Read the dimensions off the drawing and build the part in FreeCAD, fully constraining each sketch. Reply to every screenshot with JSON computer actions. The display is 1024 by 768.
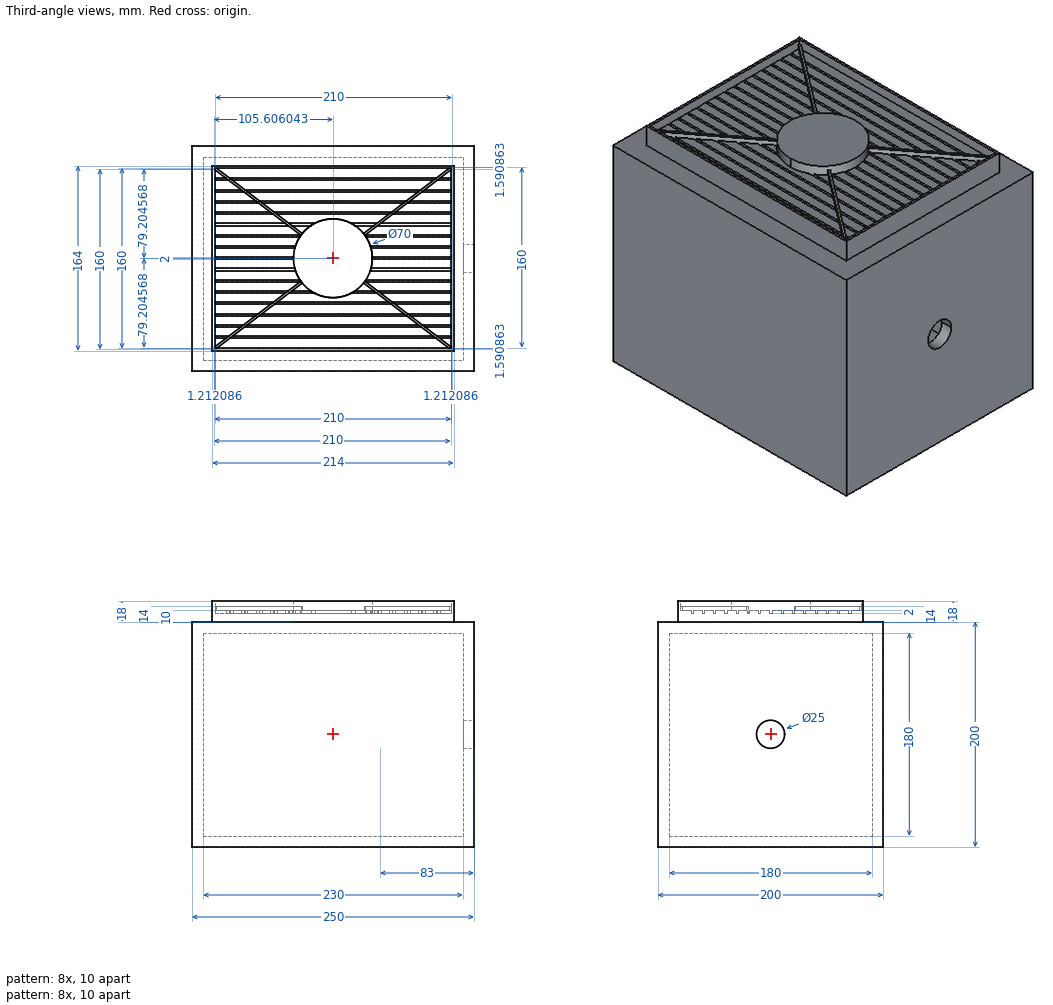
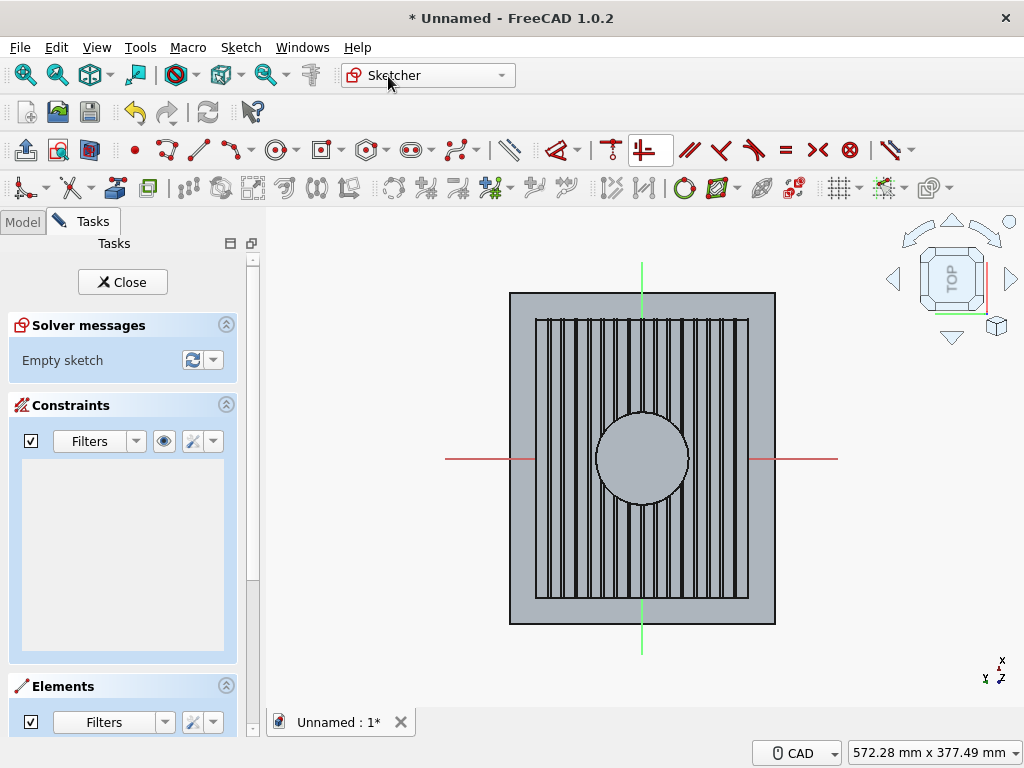
{"action": "left_click", "coordinate": [90, 150]}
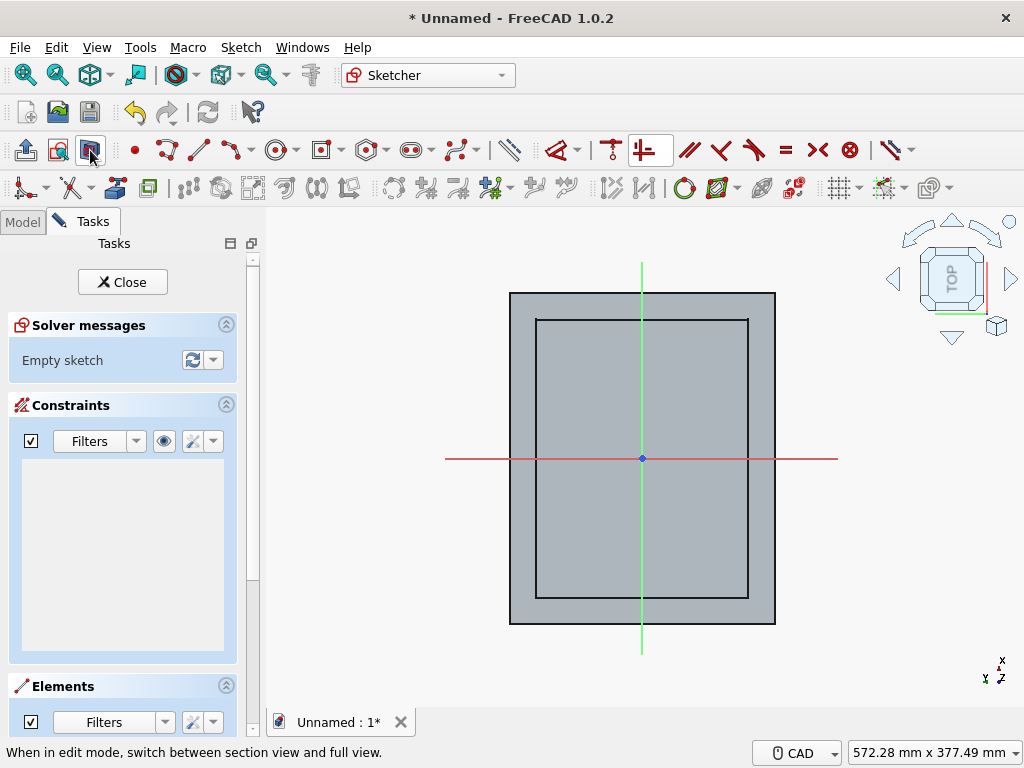
{"action": "left_click", "coordinate": [168, 150]}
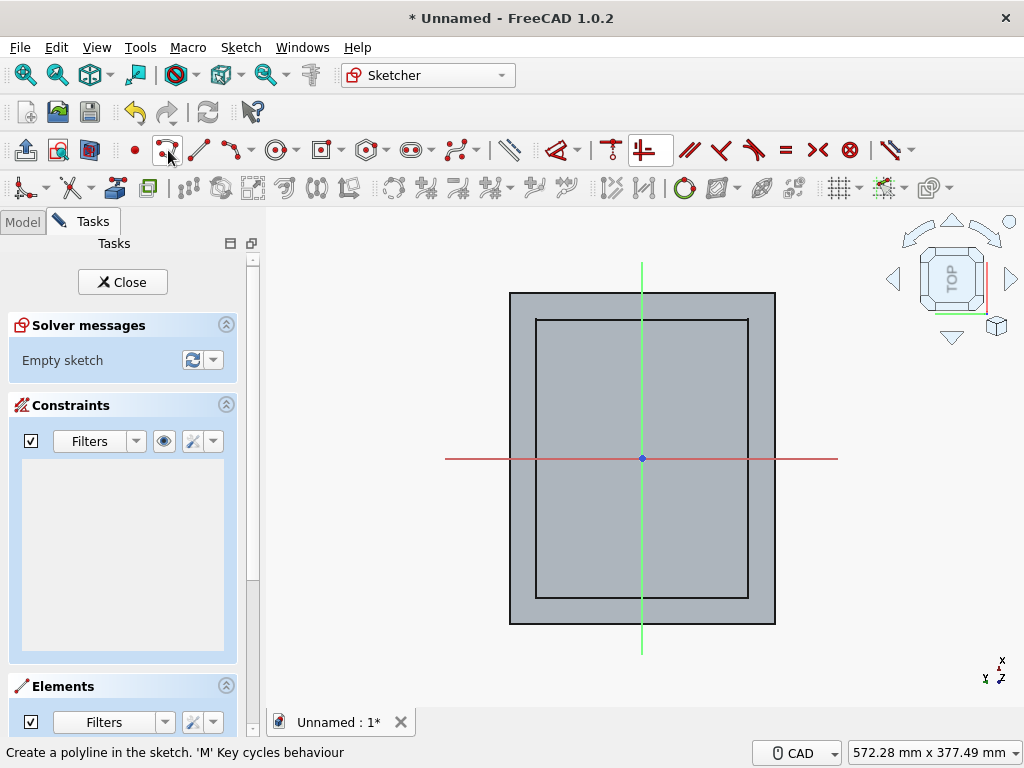
{"action": "left_click", "coordinate": [537, 598]}
{"action": "left_click", "coordinate": [749, 320]}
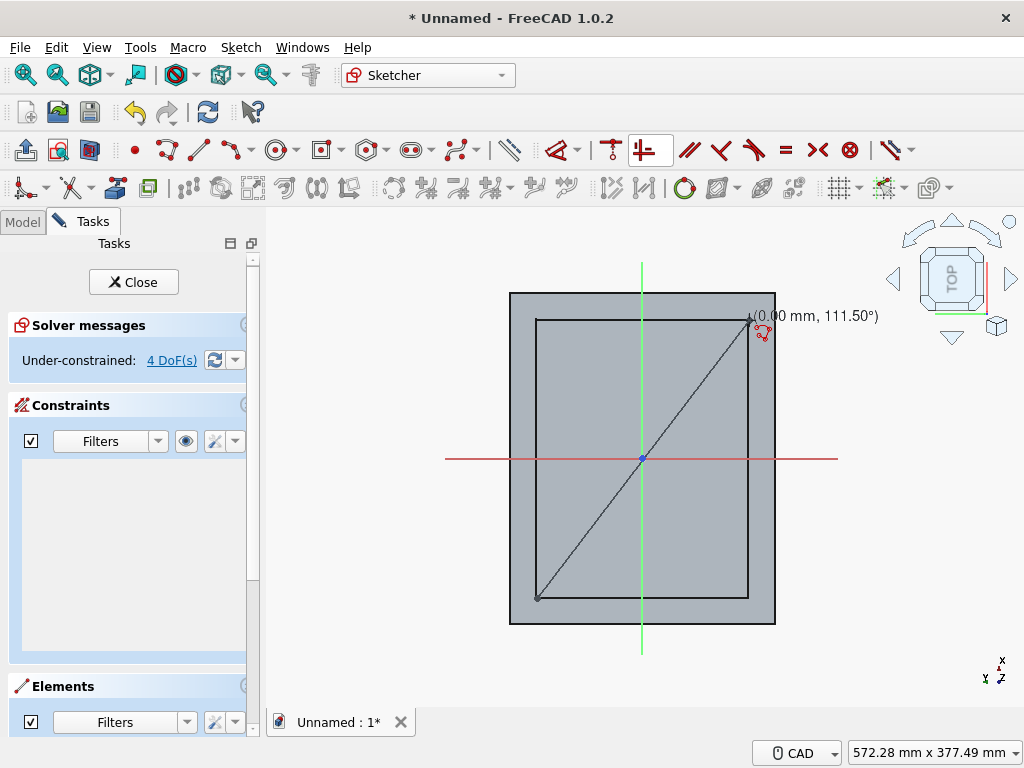
{"action": "scroll", "coordinate": [747, 319], "scroll_direction": "up", "scroll_amount": 9}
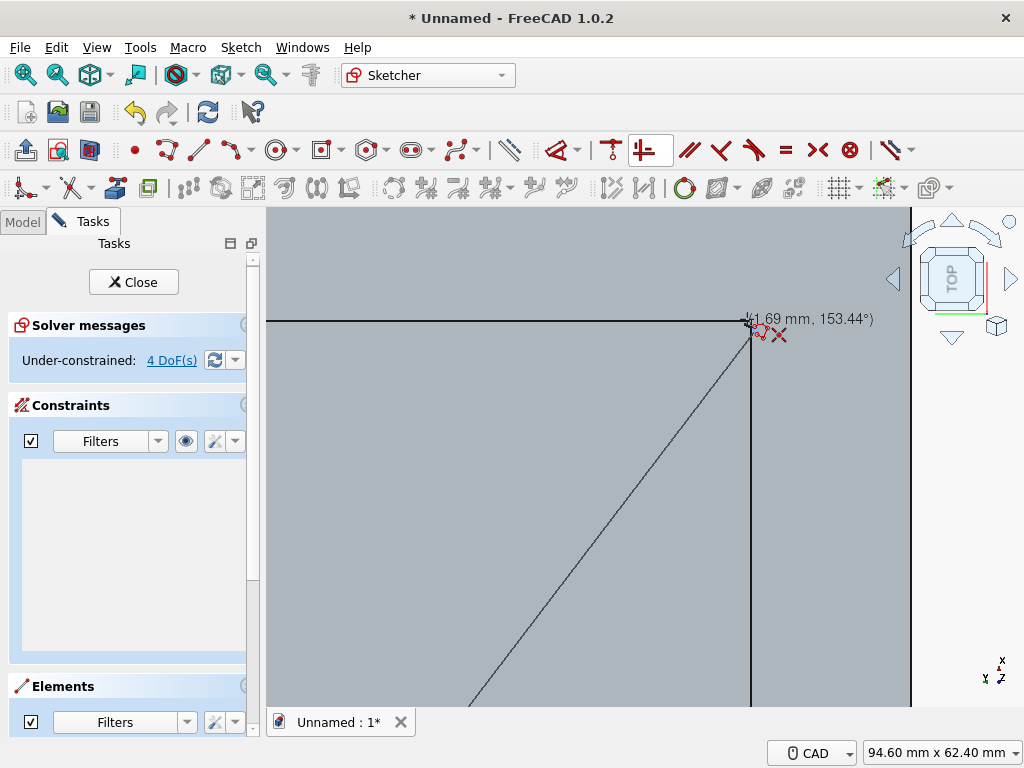
{"action": "left_click", "coordinate": [745, 316]}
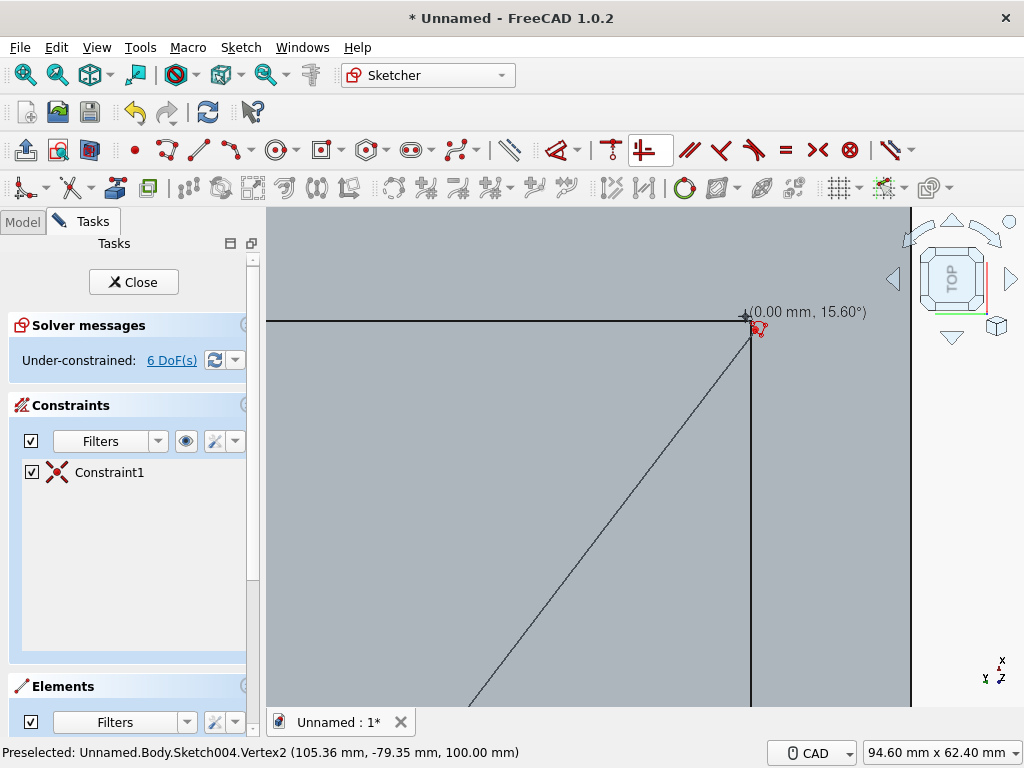
{"action": "scroll", "coordinate": [694, 279], "scroll_direction": "down", "scroll_amount": 8}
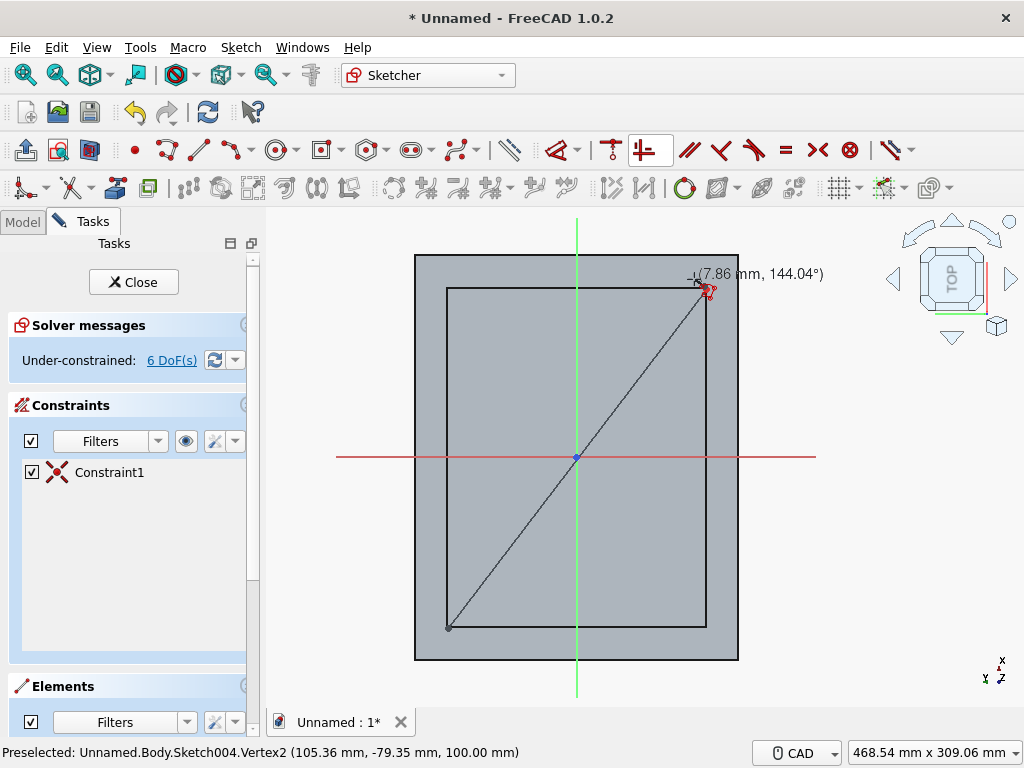
{"action": "scroll", "coordinate": [446, 626], "scroll_direction": "up", "scroll_amount": 8}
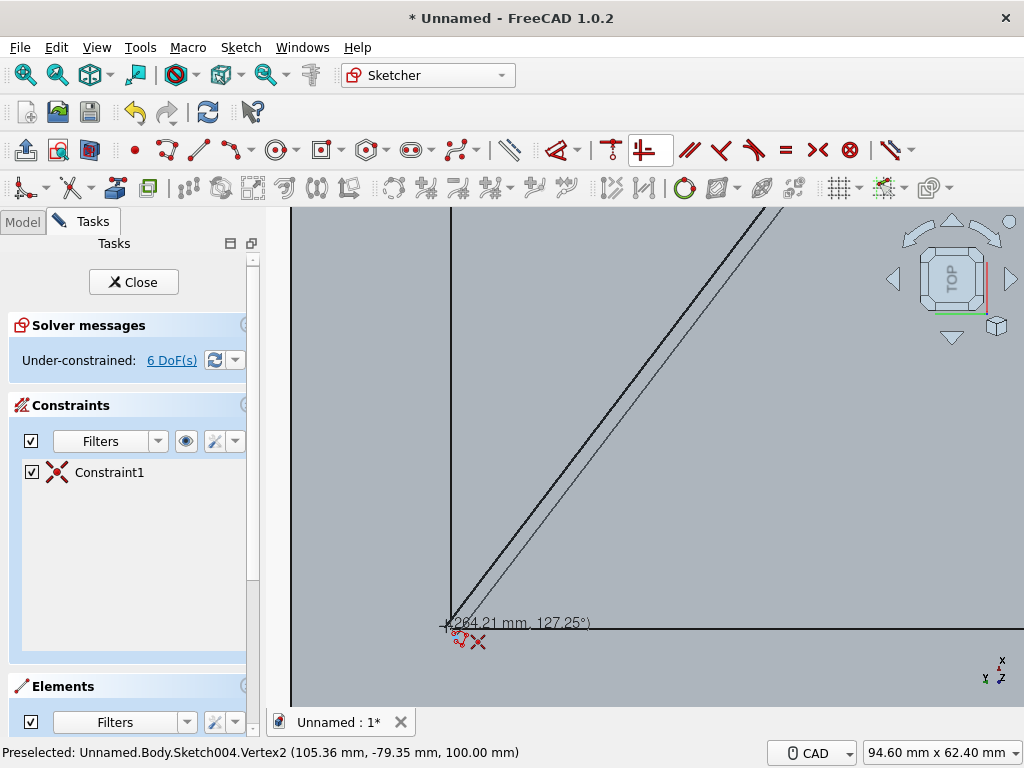
{"action": "left_click", "coordinate": [444, 624]}
{"action": "left_click", "coordinate": [455, 637]}
{"action": "key", "text": "Escape"}
{"action": "key", "text": "Escape"}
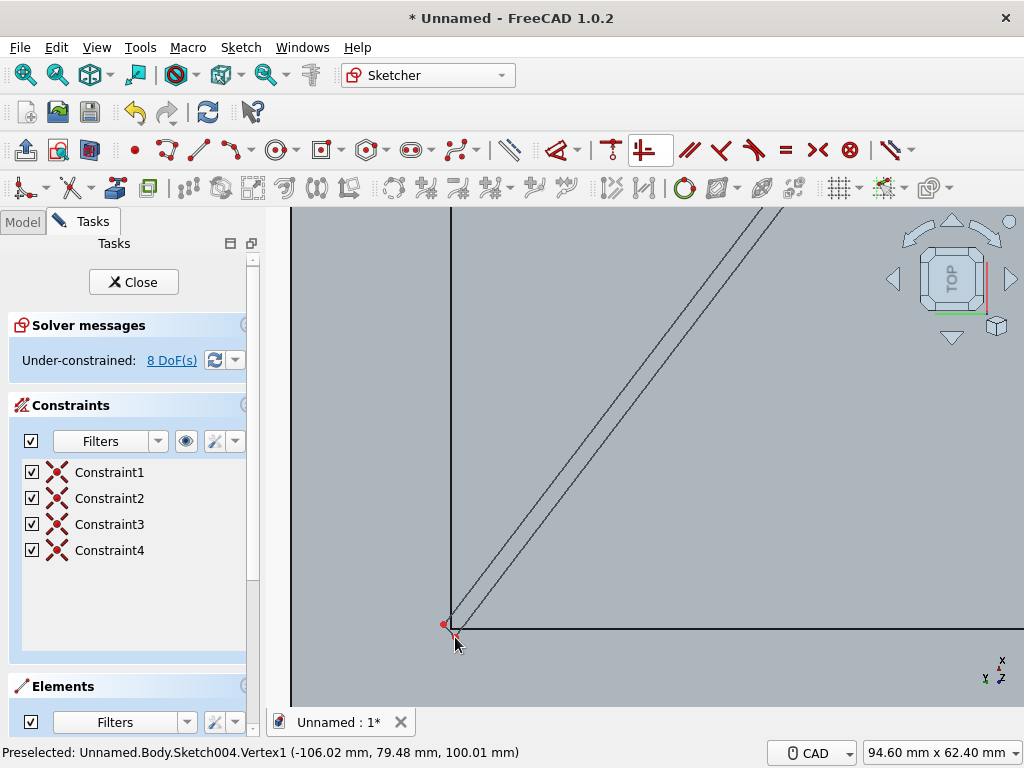
{"action": "left_click", "coordinate": [556, 150]}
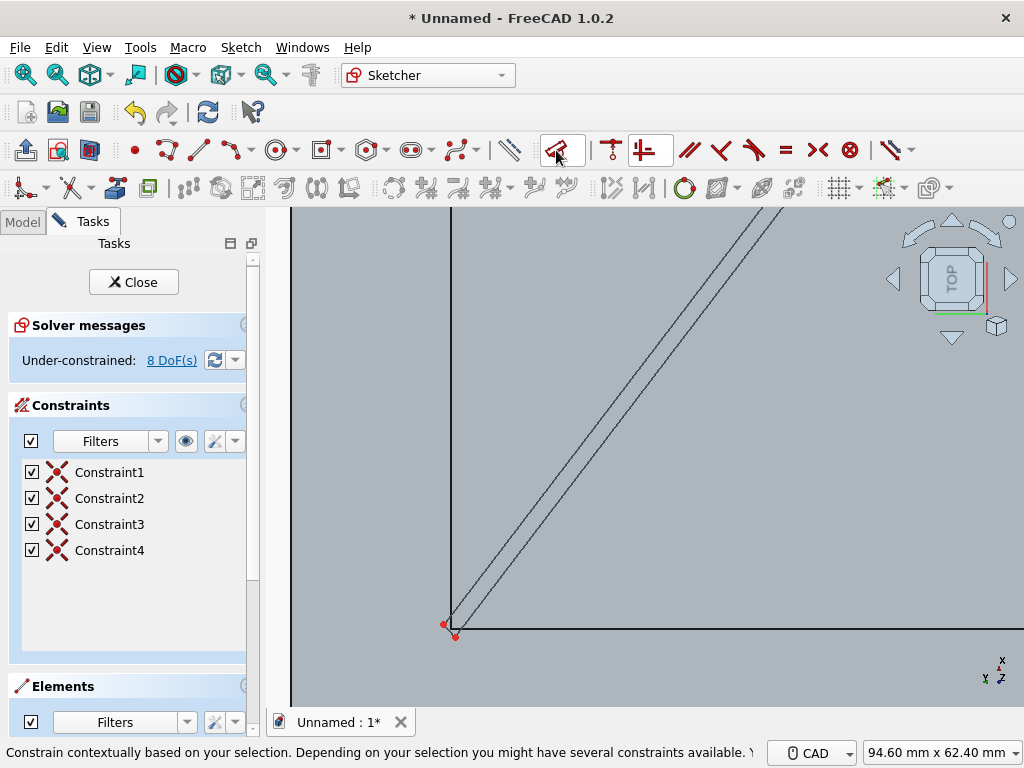
{"action": "left_click", "coordinate": [712, 301]}
{"action": "left_click", "coordinate": [657, 671]}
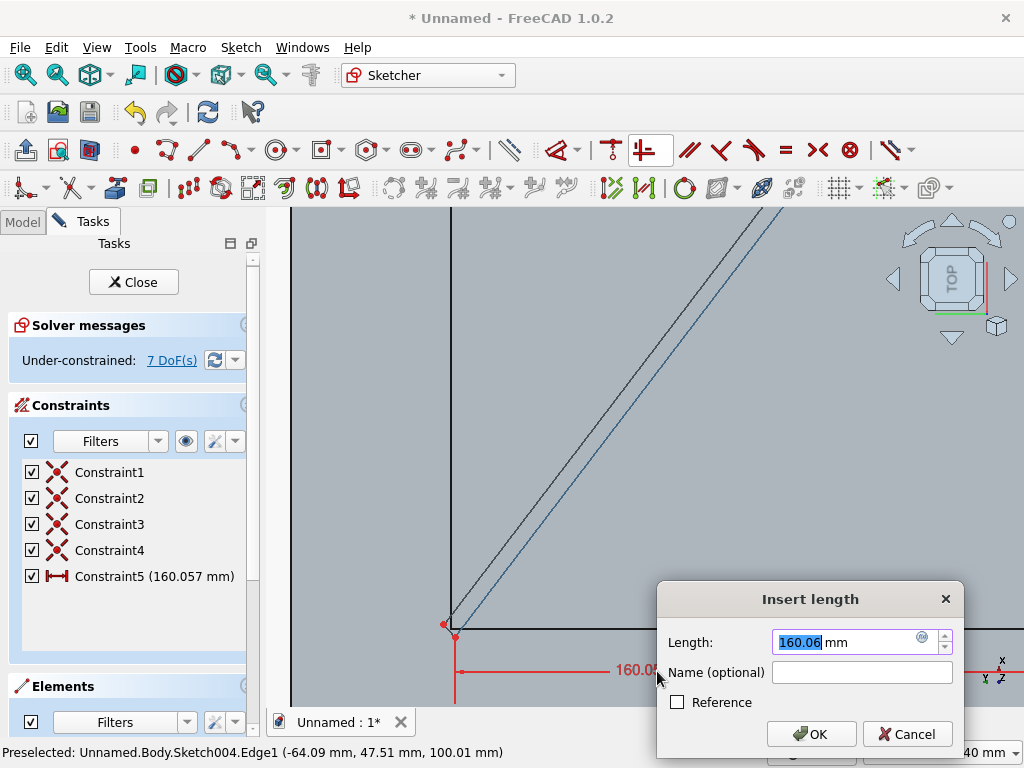
{"action": "type", "text": "160"}
{"action": "key", "text": "Return"}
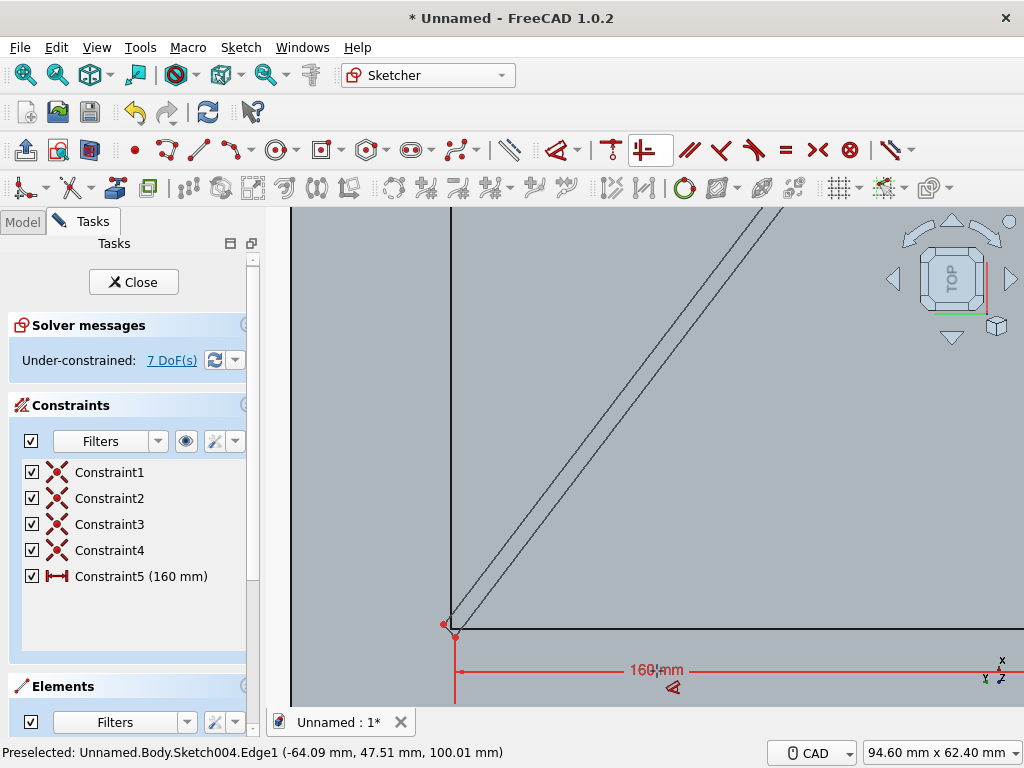
{"action": "left_click", "coordinate": [711, 301]}
{"action": "left_click", "coordinate": [421, 436]}